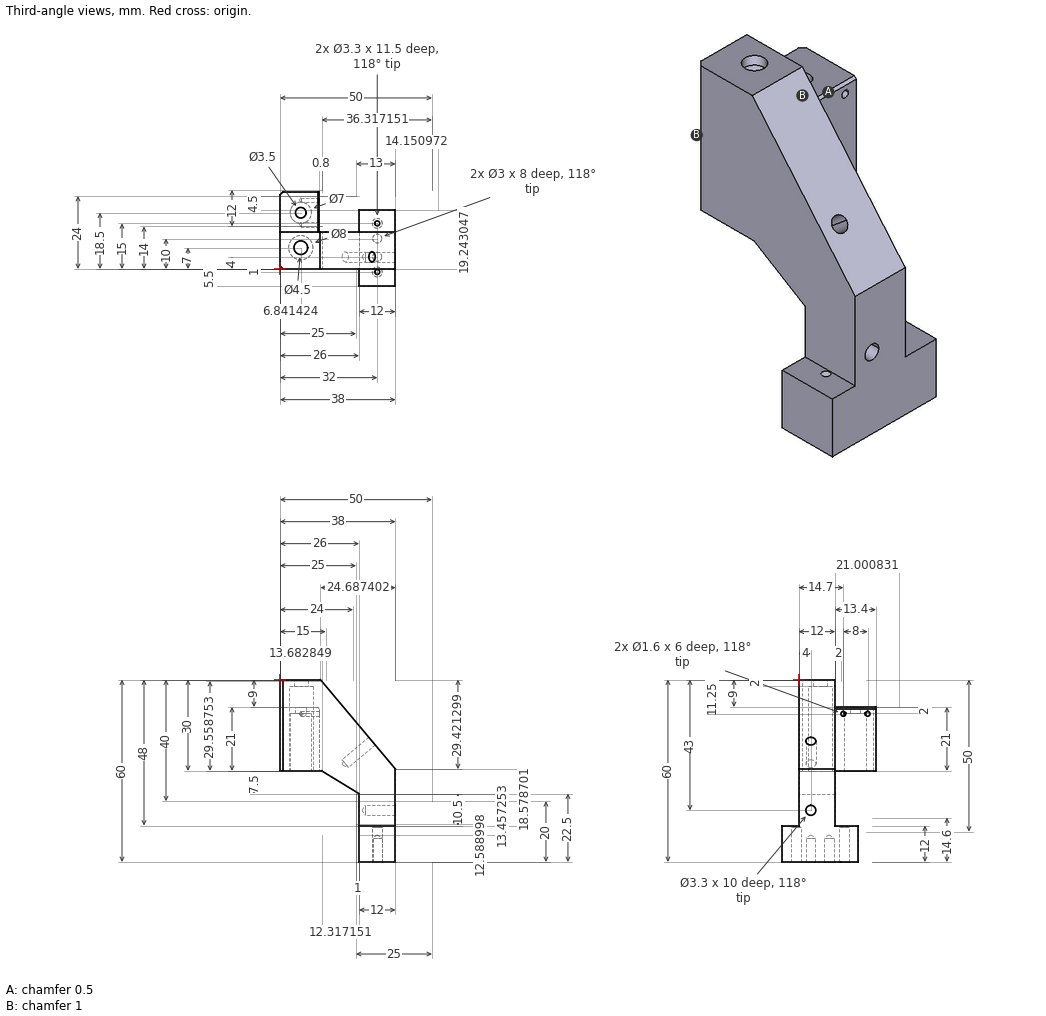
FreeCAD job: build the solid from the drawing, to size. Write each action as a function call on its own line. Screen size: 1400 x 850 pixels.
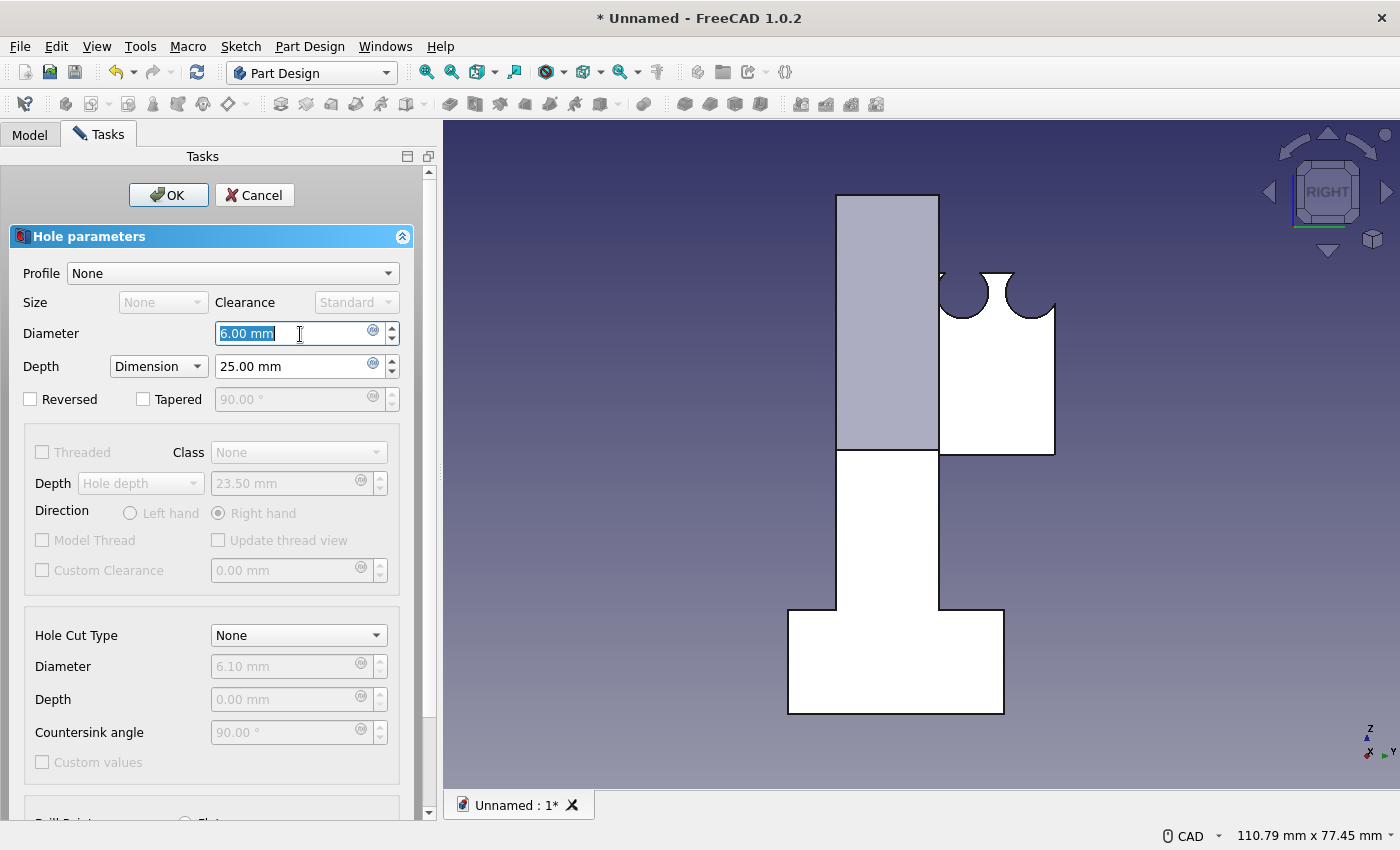
text(1.6)
key(Tab)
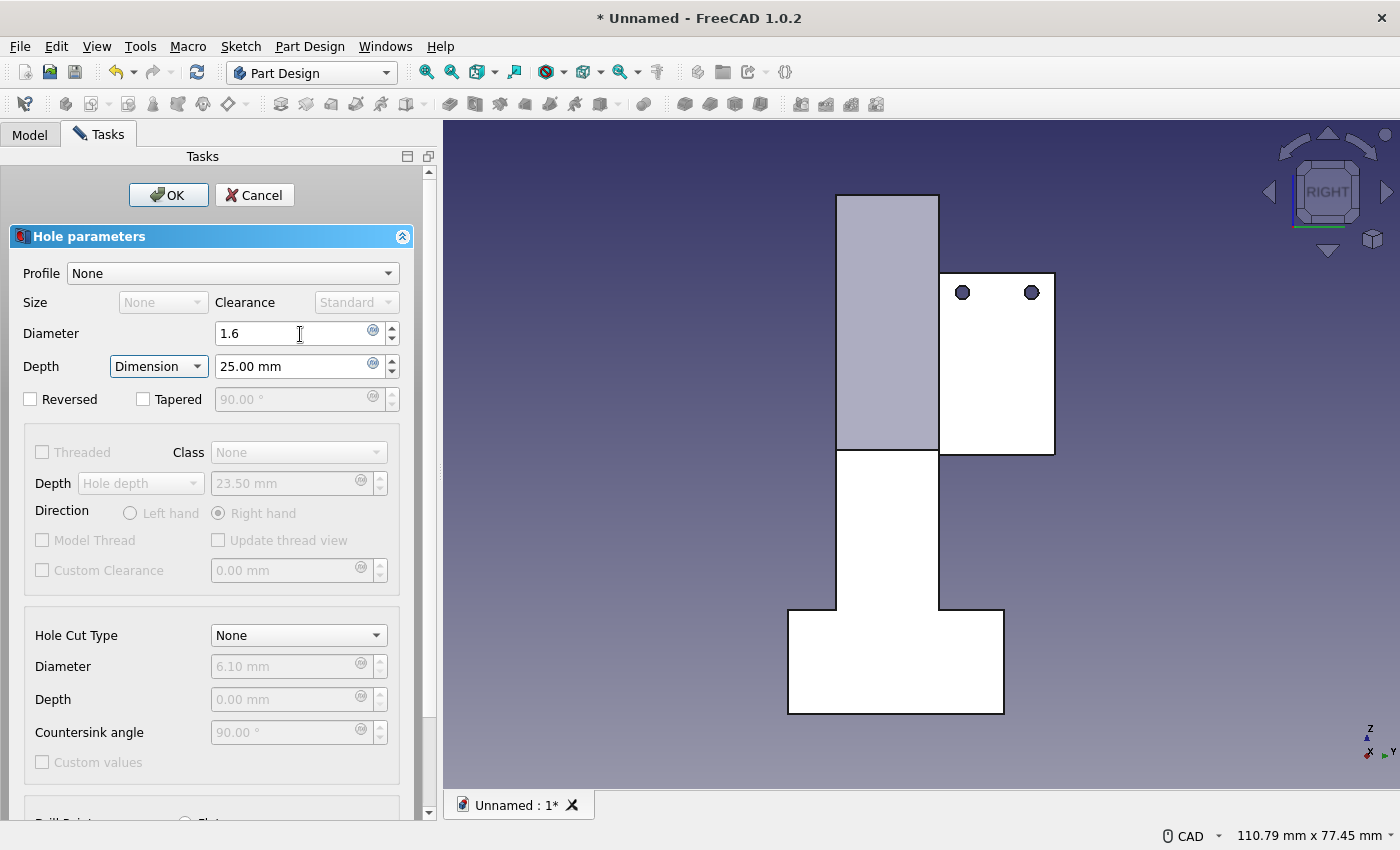
triple_click(300, 366)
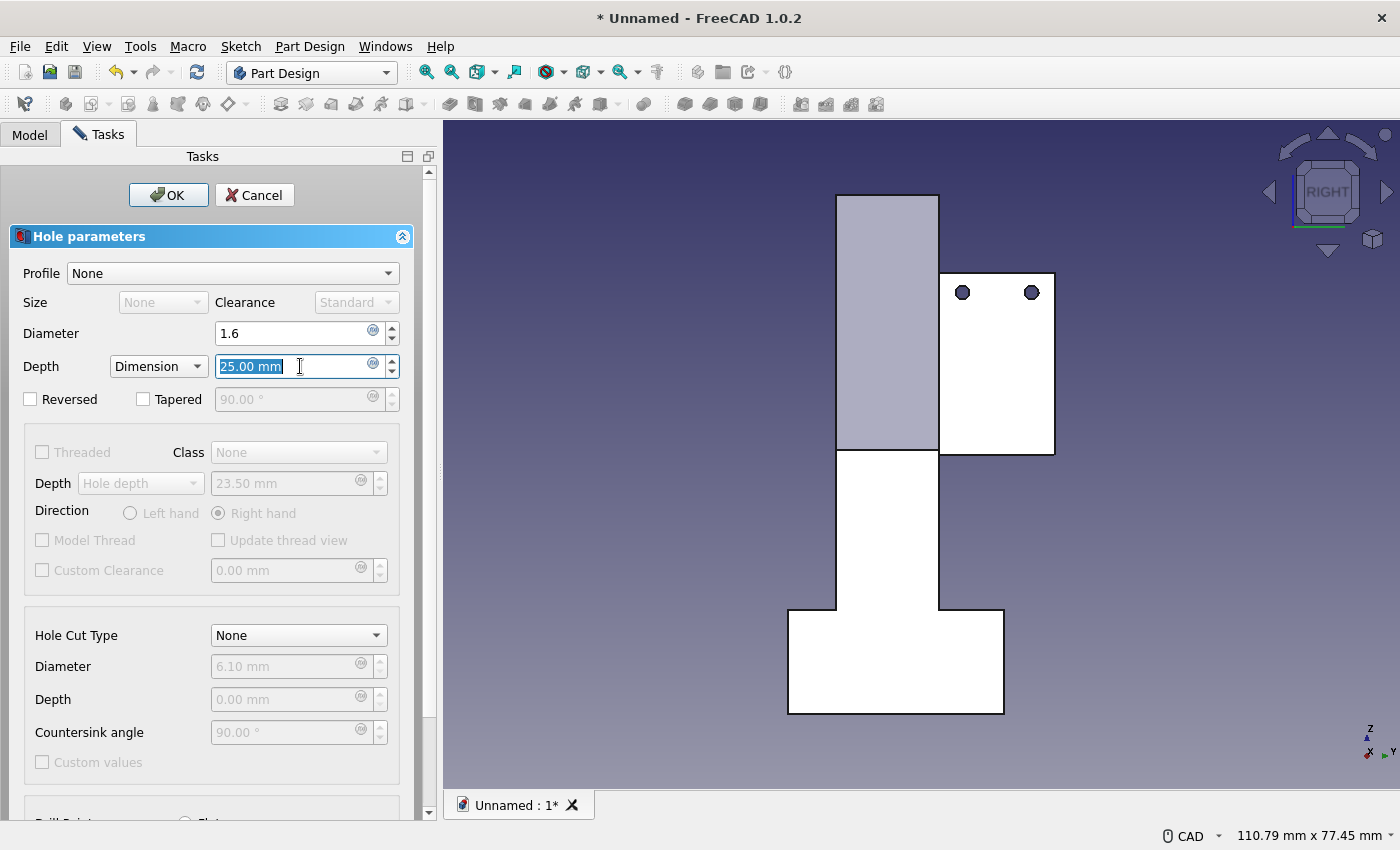
text(6)
key(Tab)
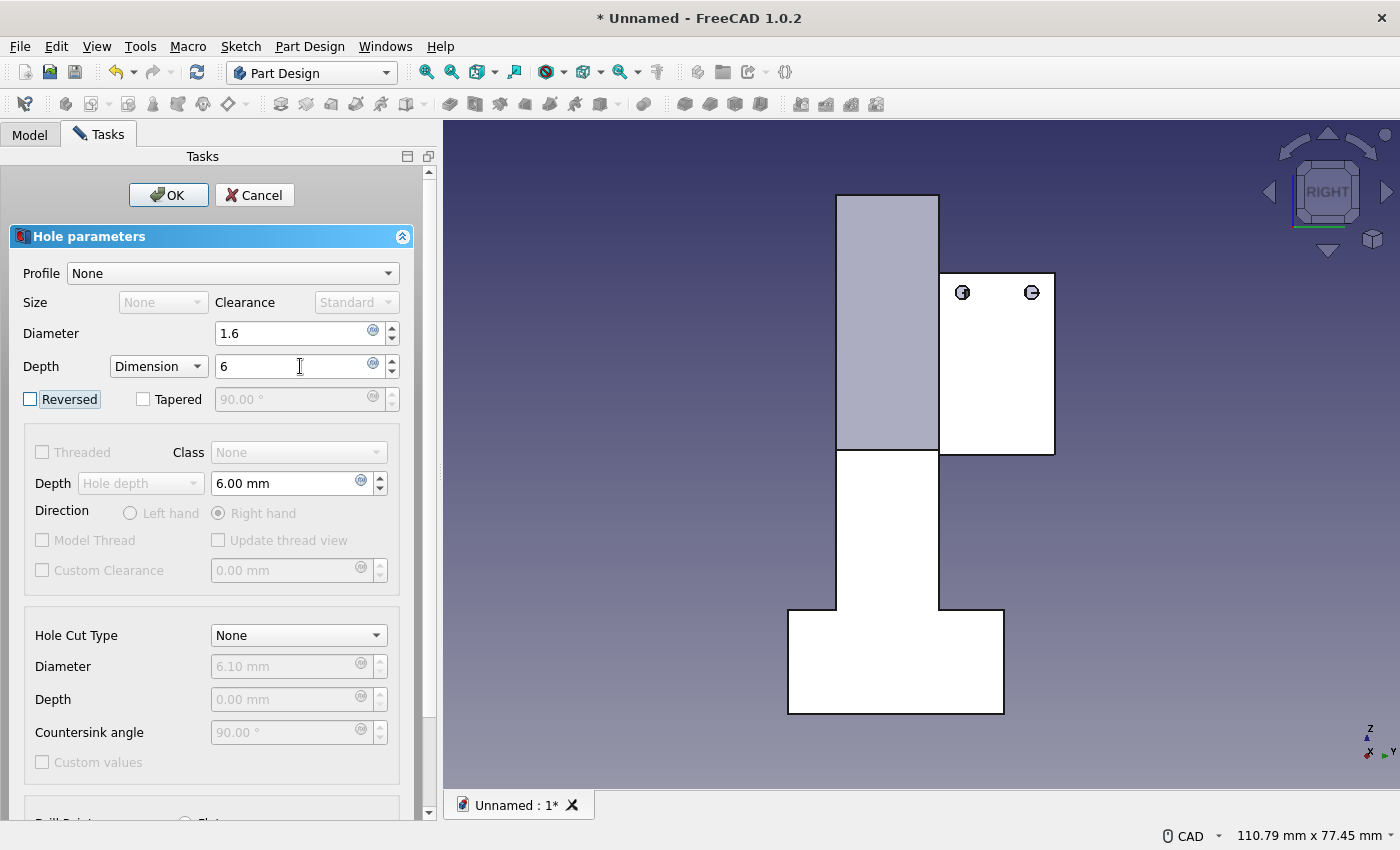
click(169, 195)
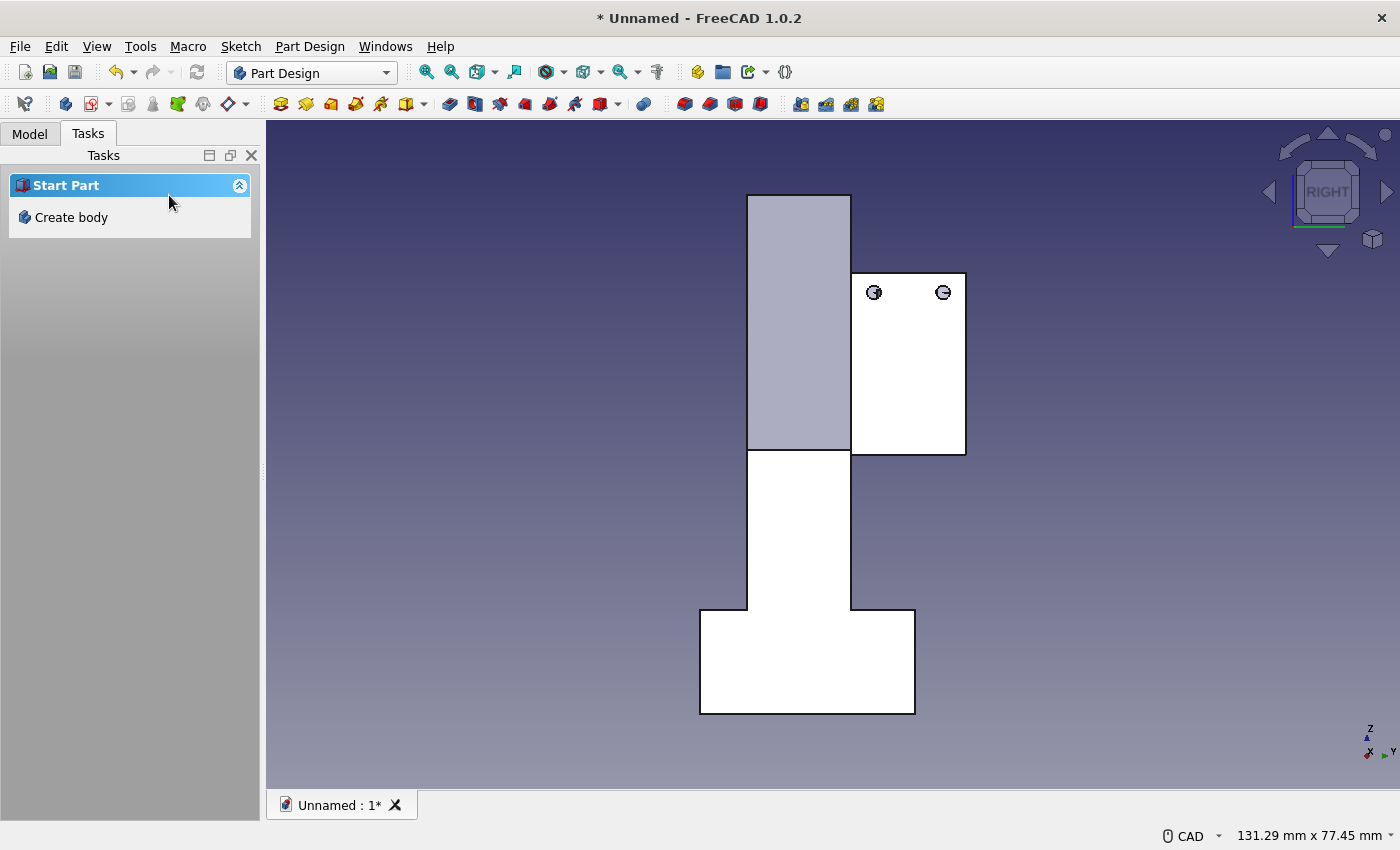
key(5)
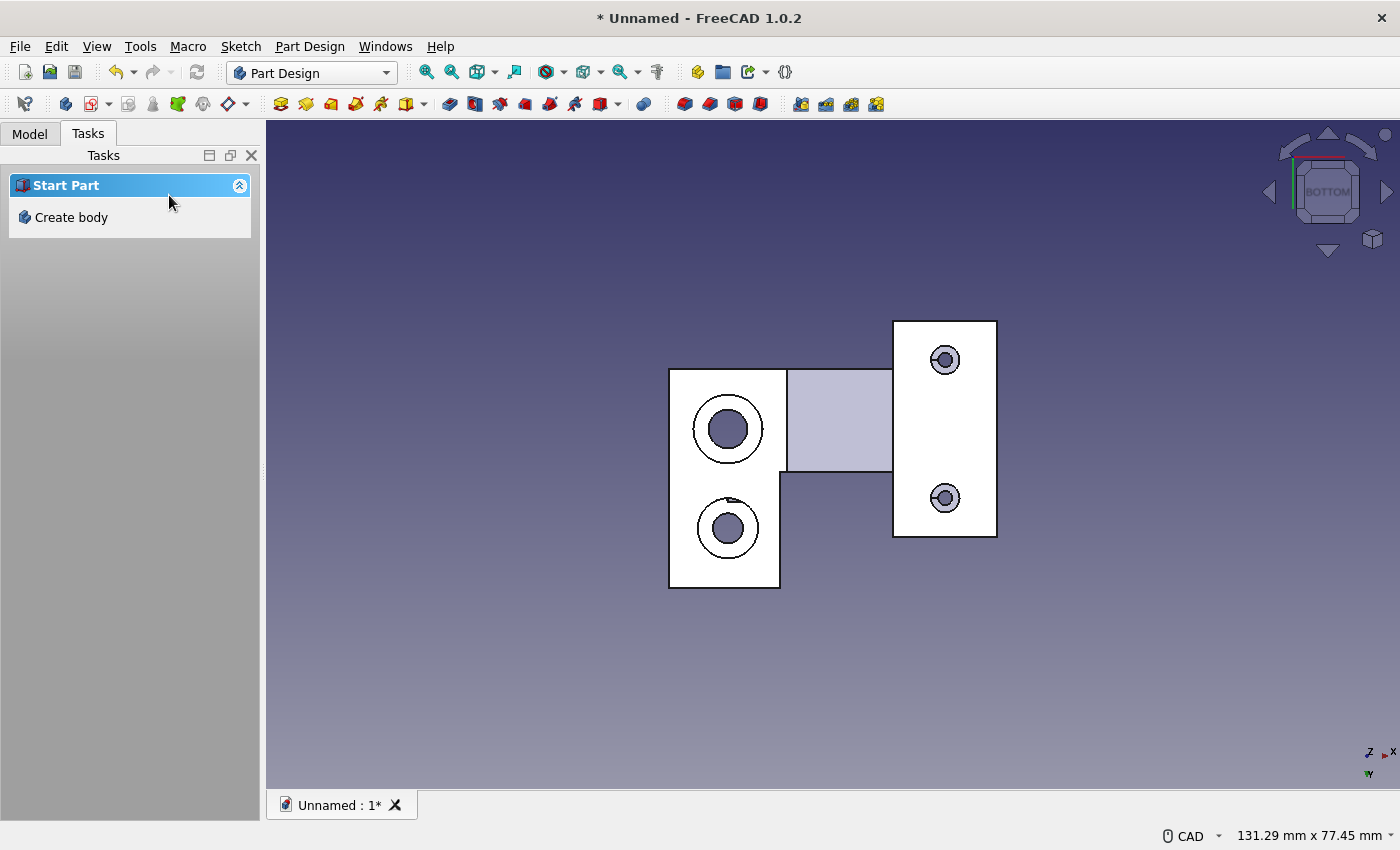
click(427, 72)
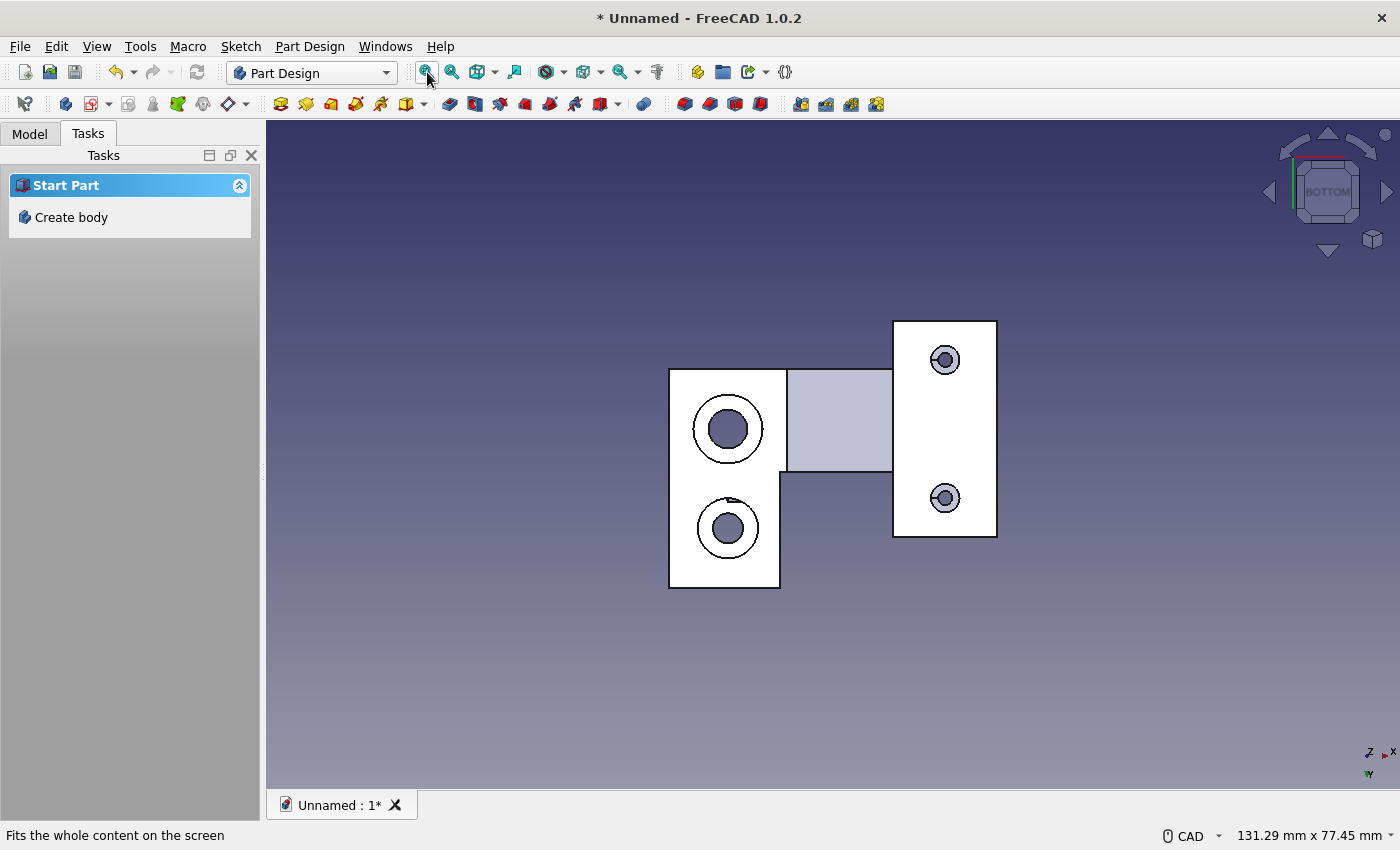
click(945, 428)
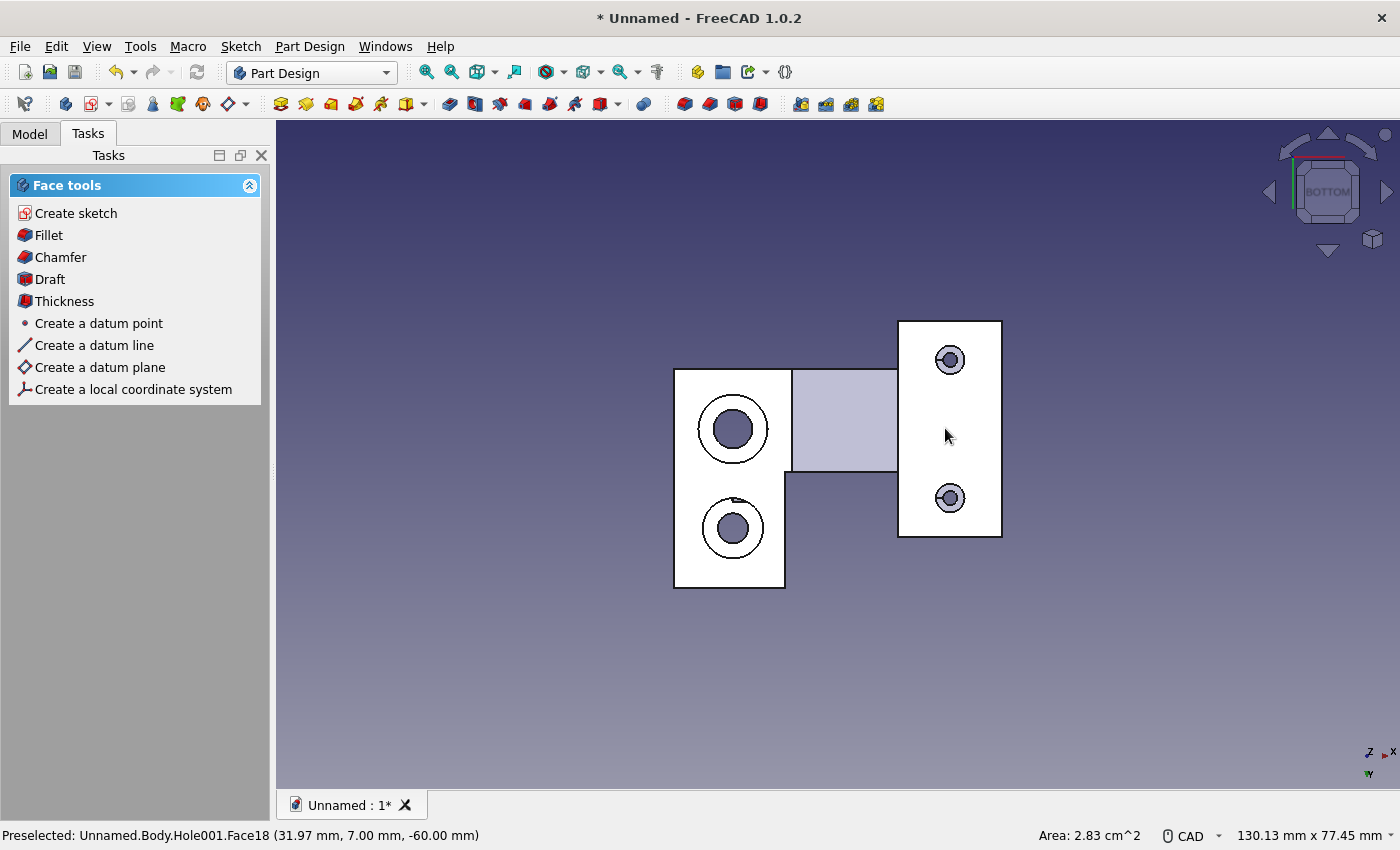
click(90, 104)